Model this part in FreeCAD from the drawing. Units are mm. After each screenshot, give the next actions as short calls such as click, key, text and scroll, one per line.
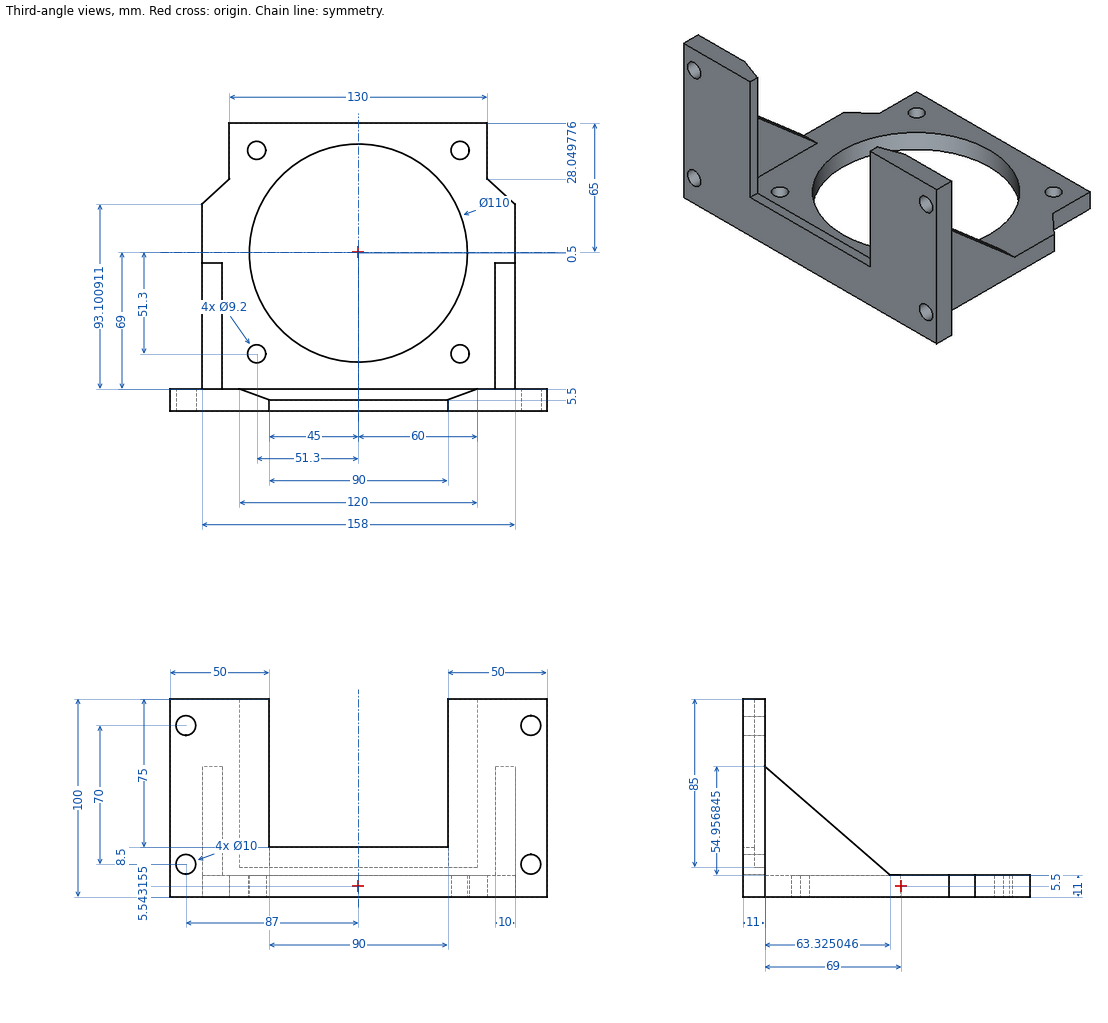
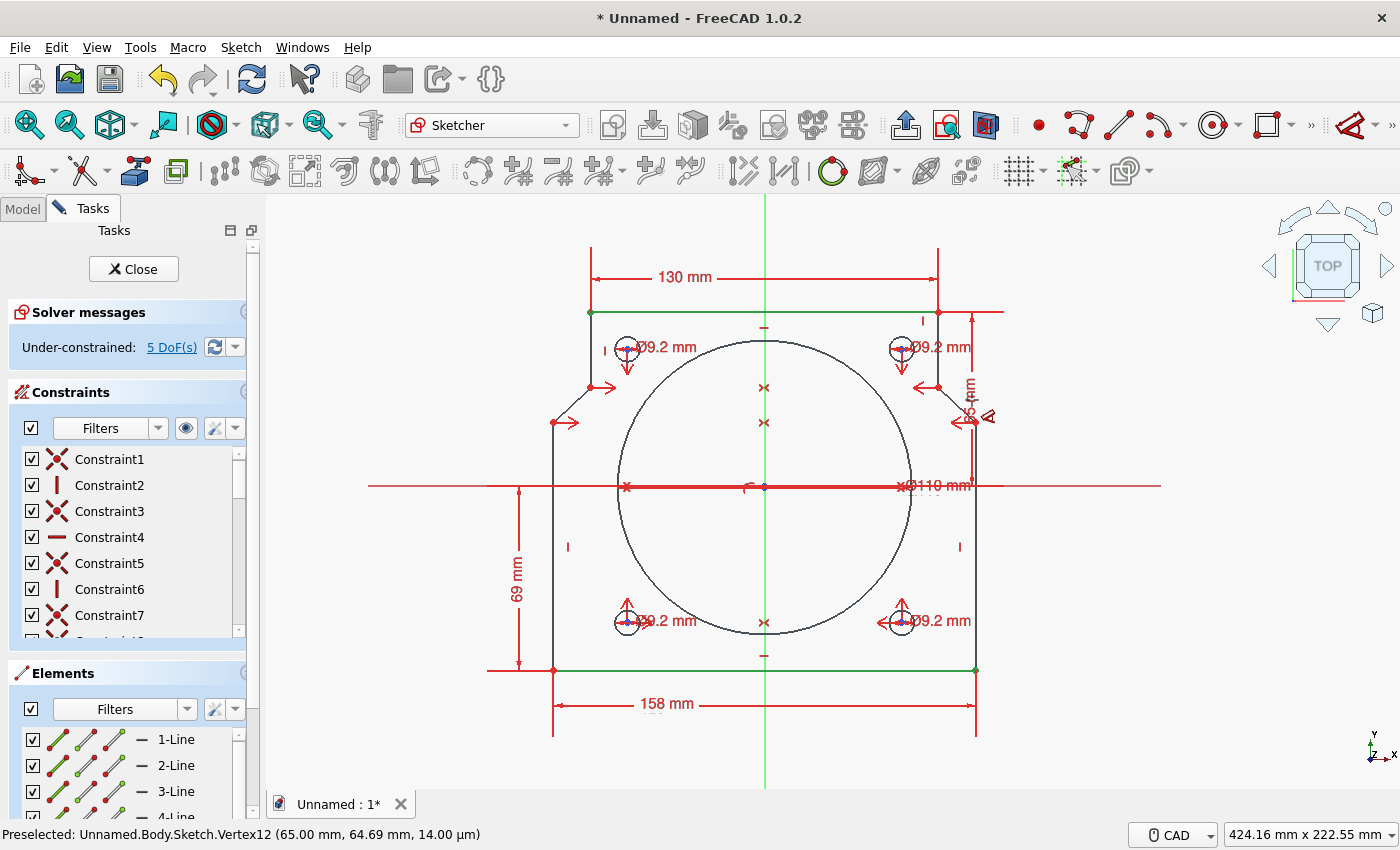
scroll(765, 488, up, 17)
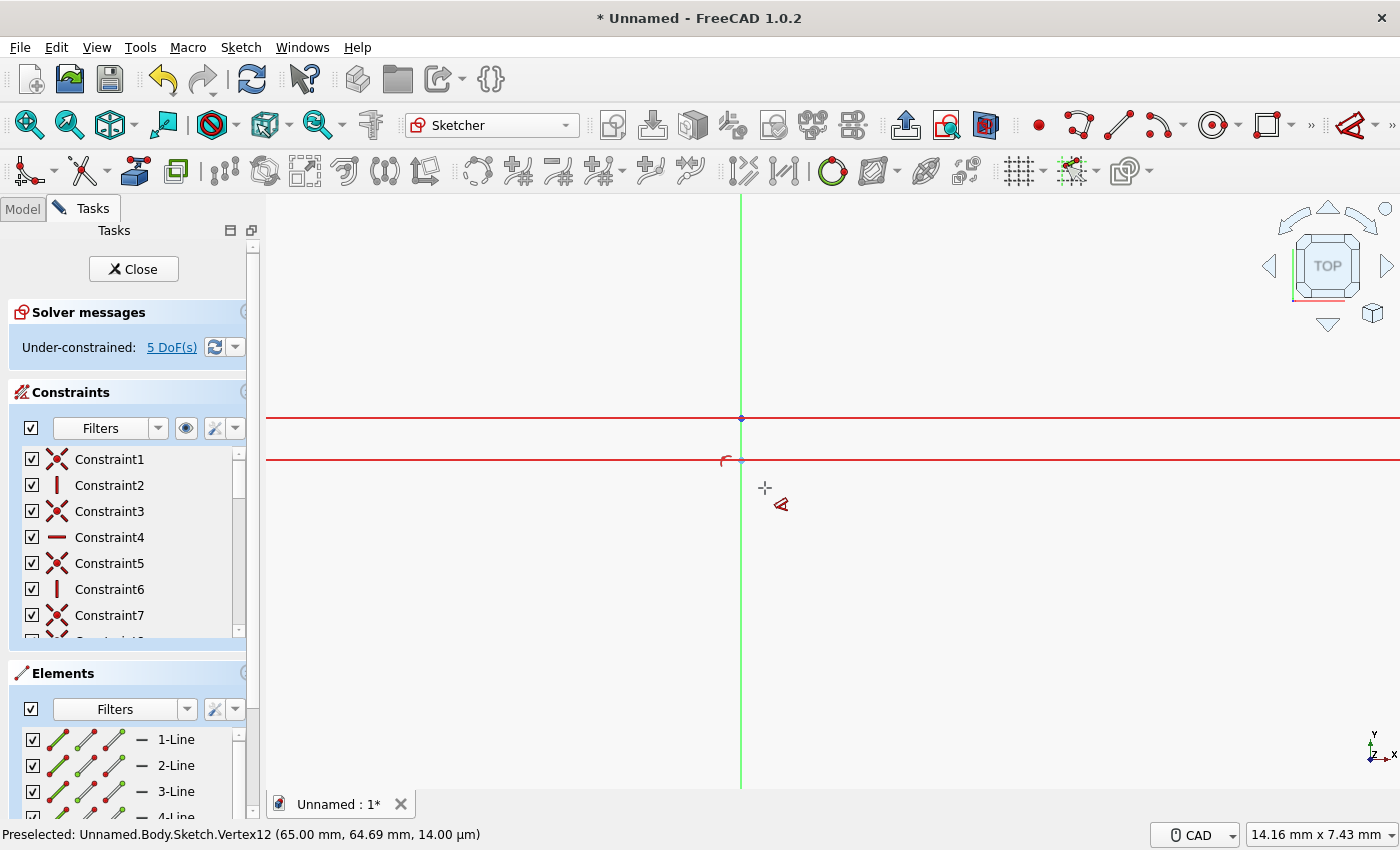
click(741, 460)
click(775, 439)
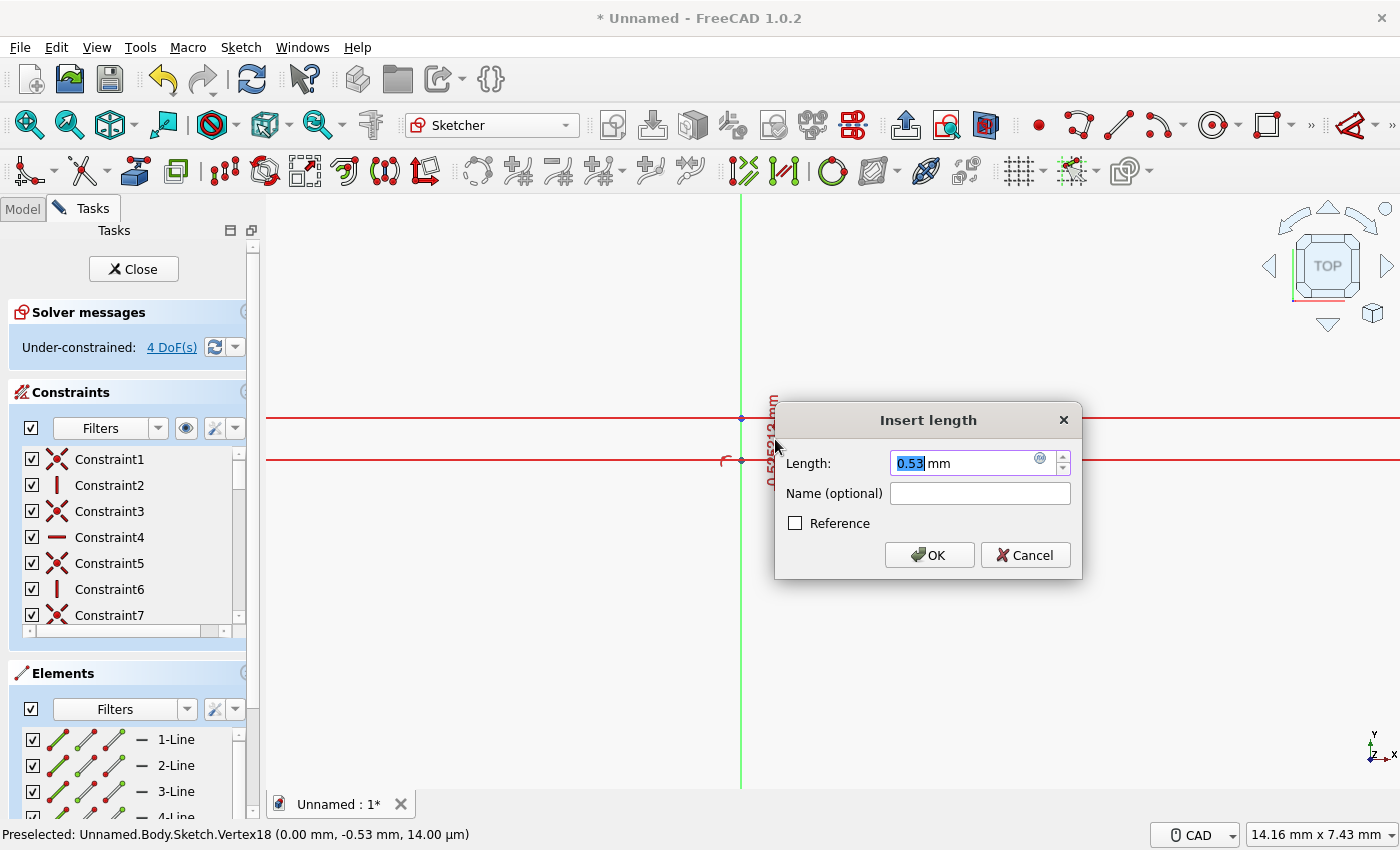
text(0.5)
key(Return)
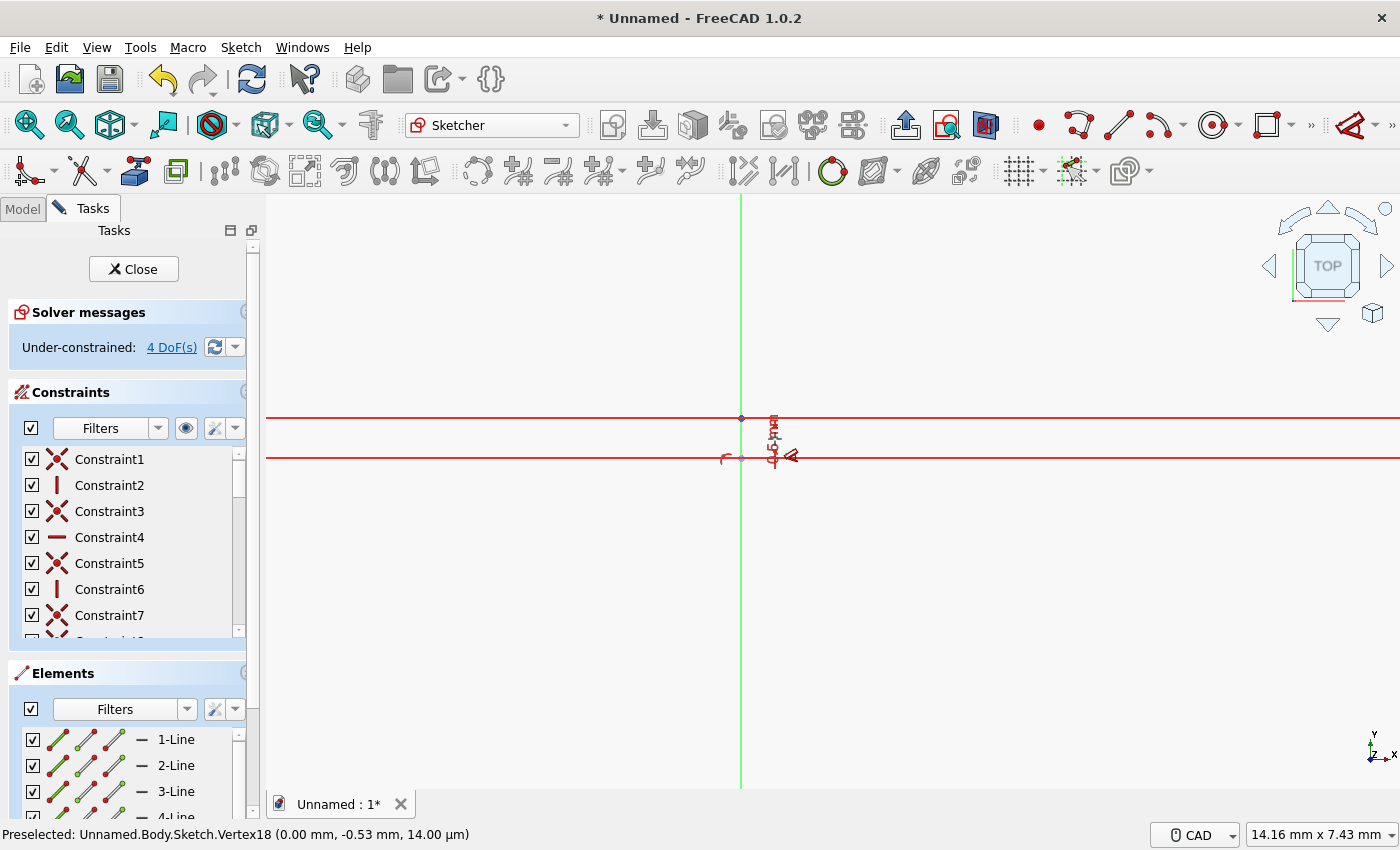
scroll(765, 488, down, 16)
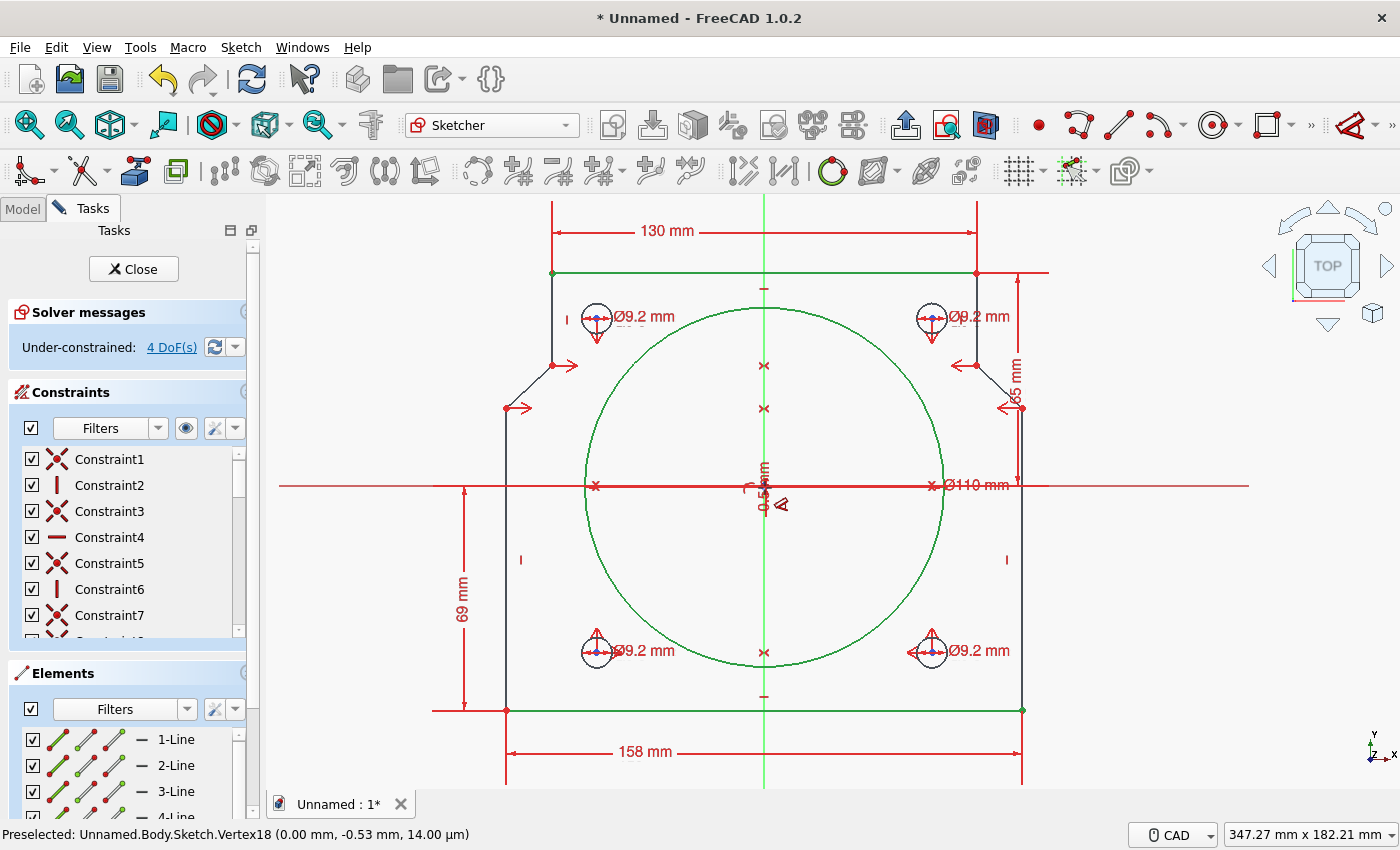
click(597, 653)
click(681, 687)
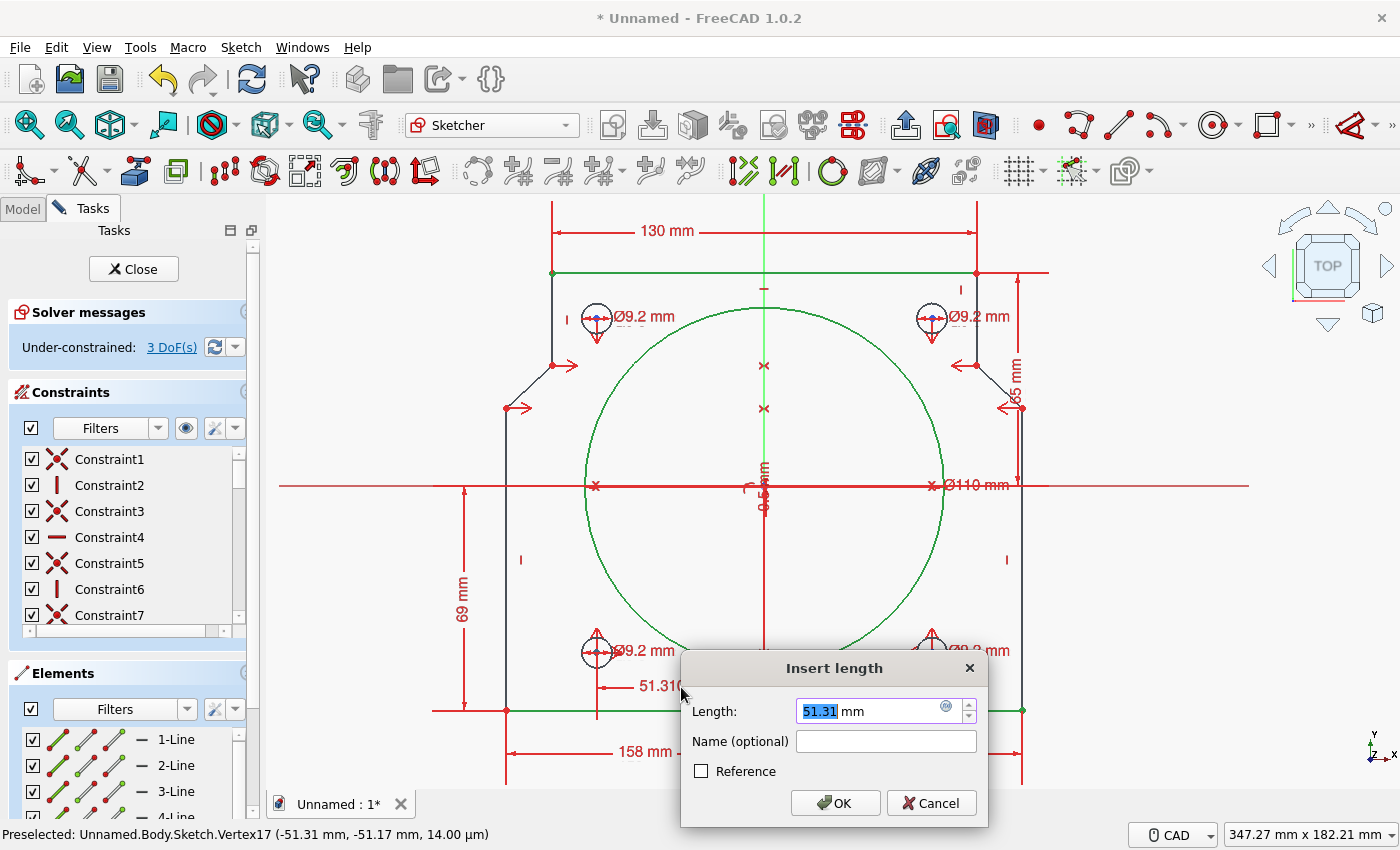
text(51.3)
key(Return)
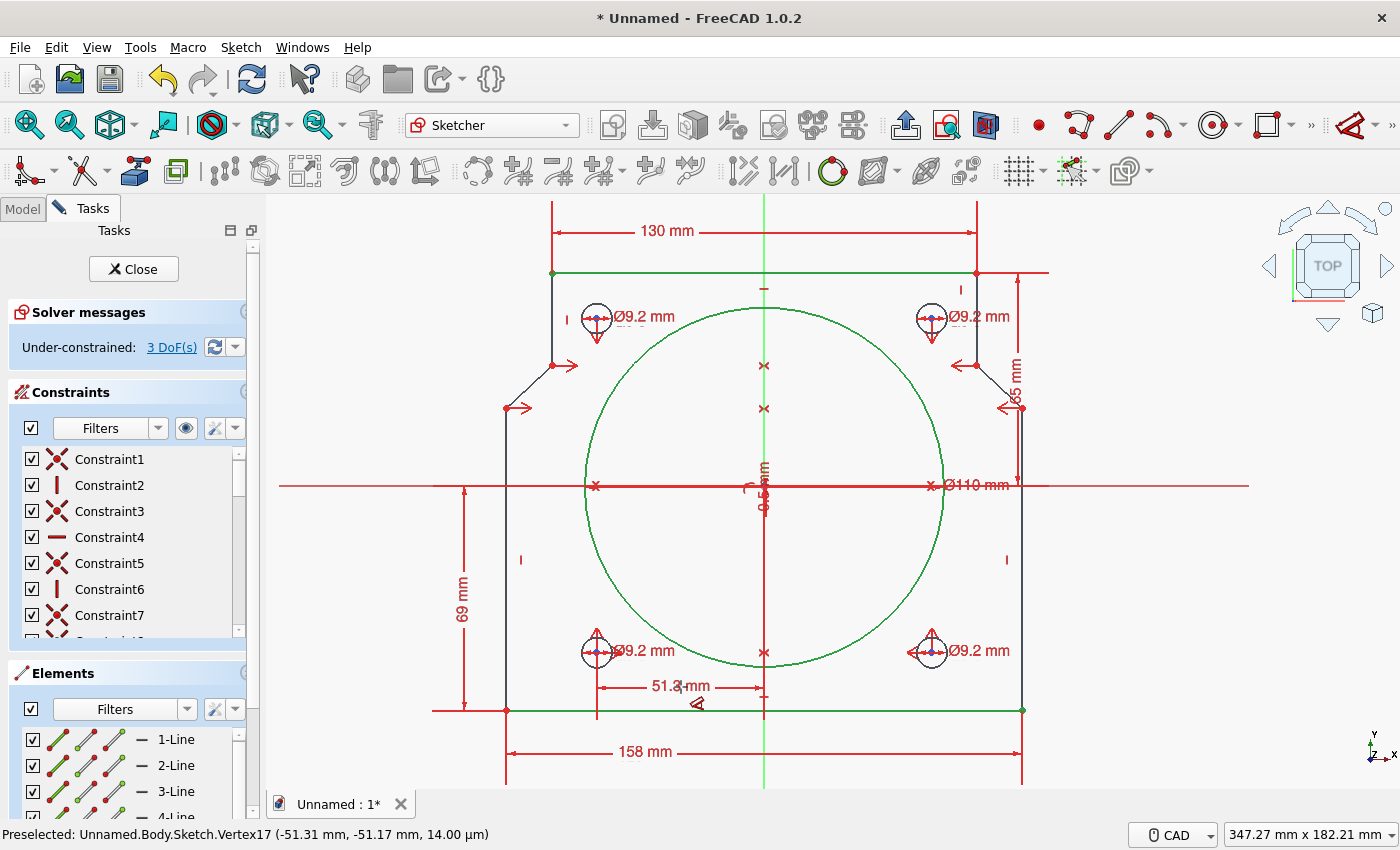
click(597, 653)
click(563, 569)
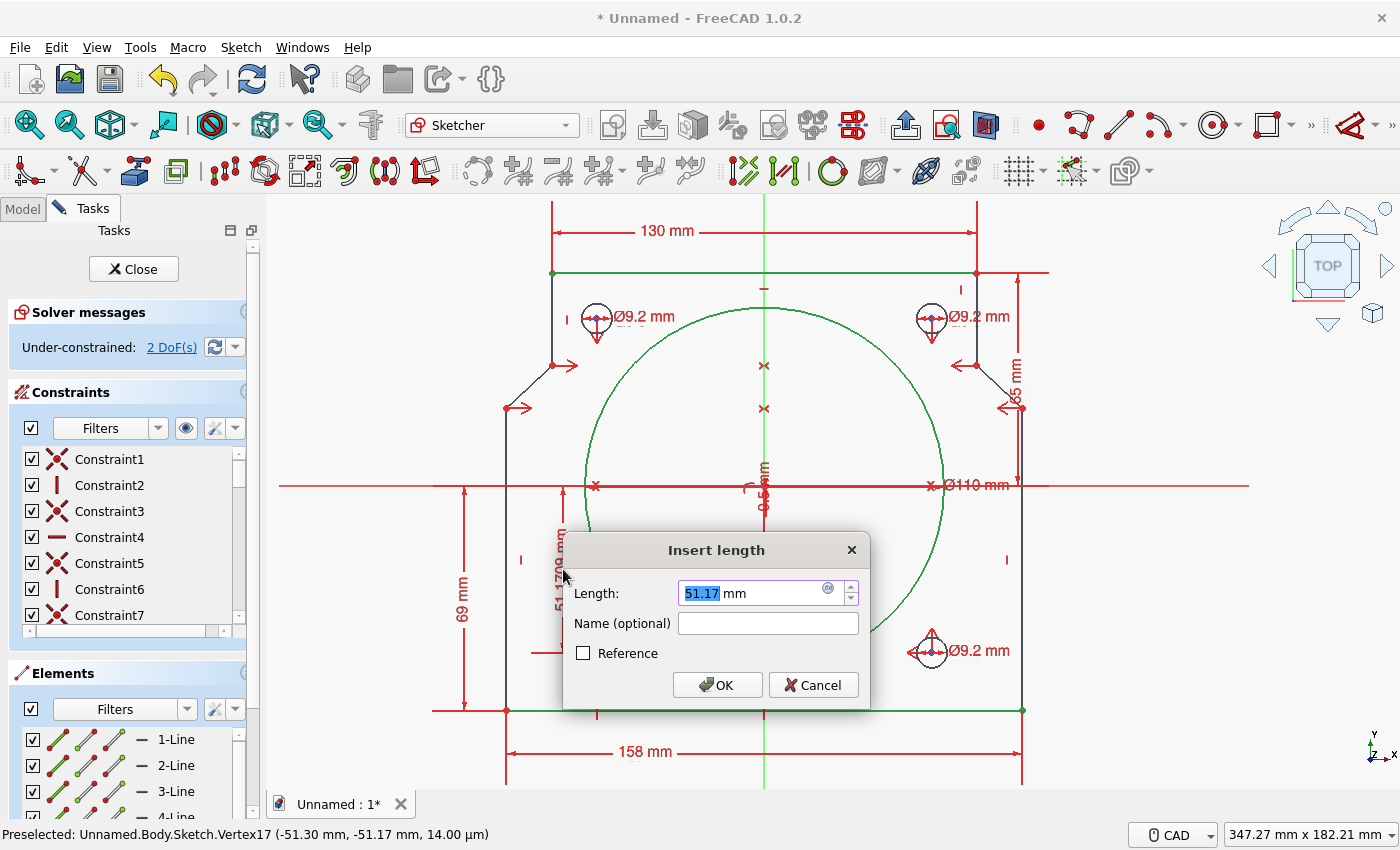
text(51.3)
key(Return)